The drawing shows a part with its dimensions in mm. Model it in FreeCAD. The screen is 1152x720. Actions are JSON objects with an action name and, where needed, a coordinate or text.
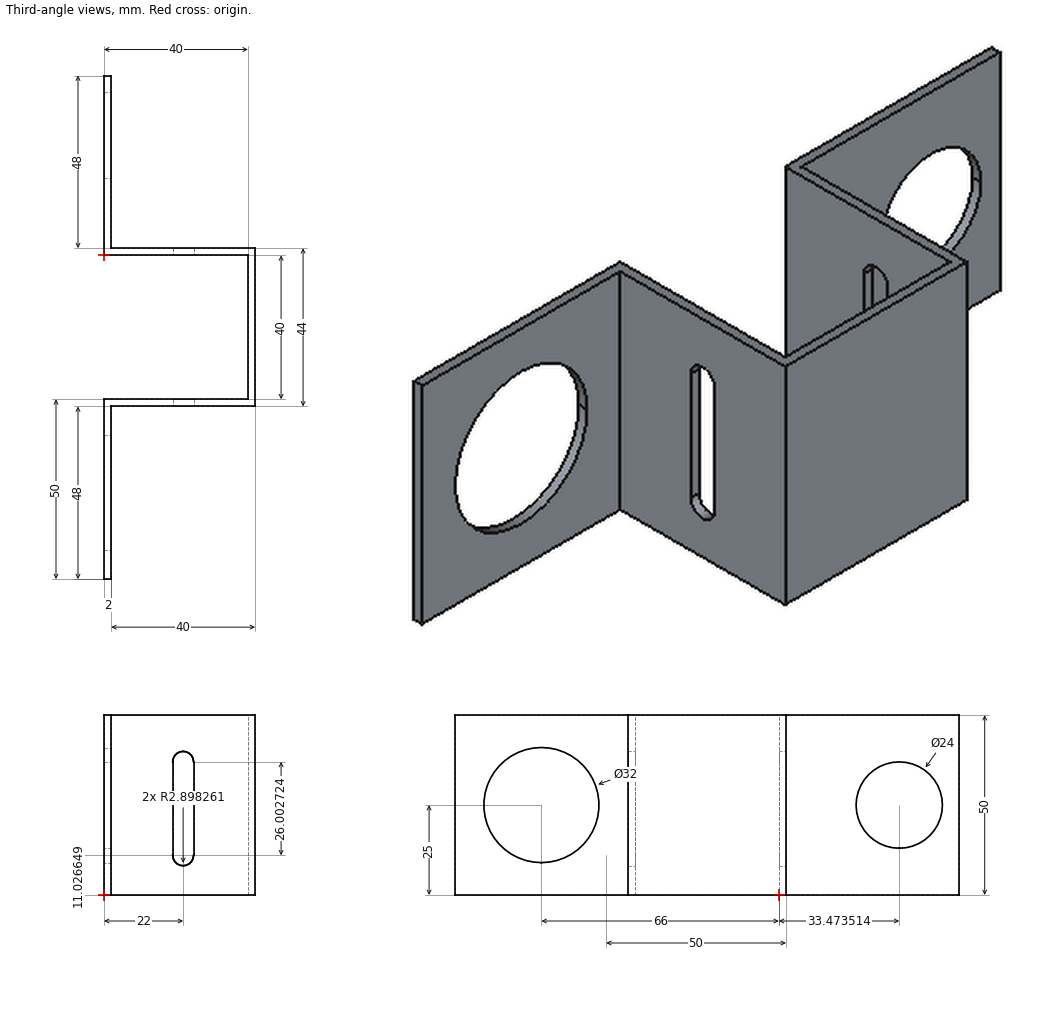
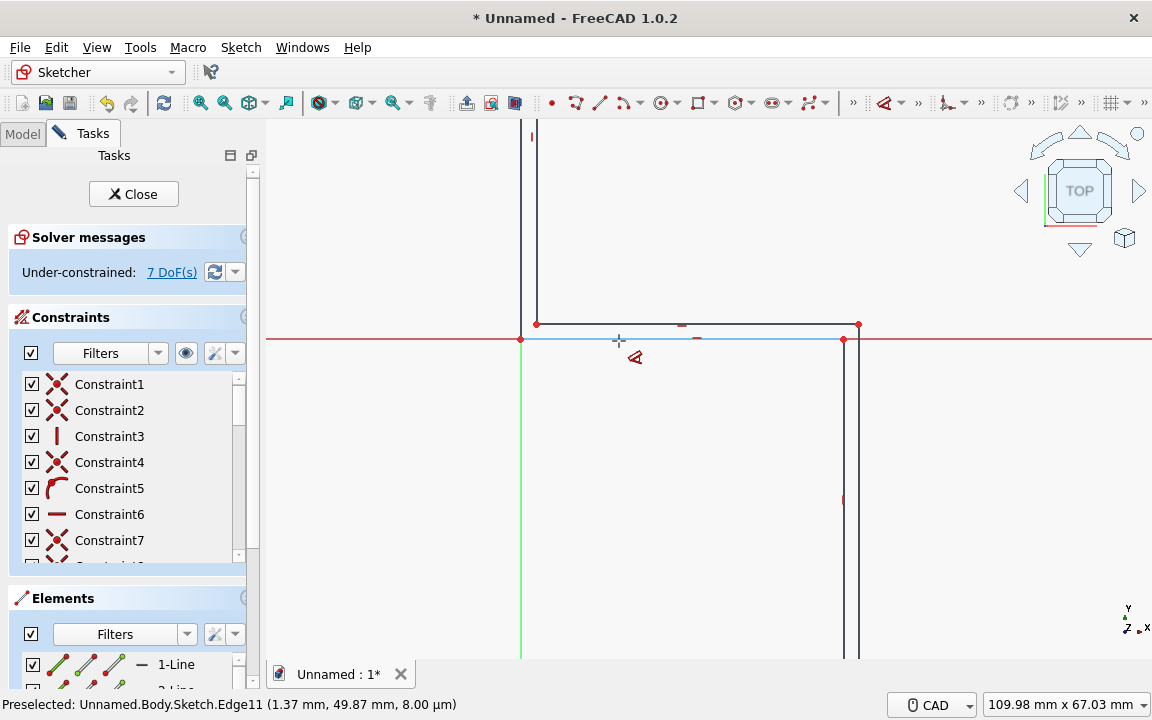
{"action": "left_click", "coordinate": [618, 339]}
{"action": "left_click", "coordinate": [682, 305]}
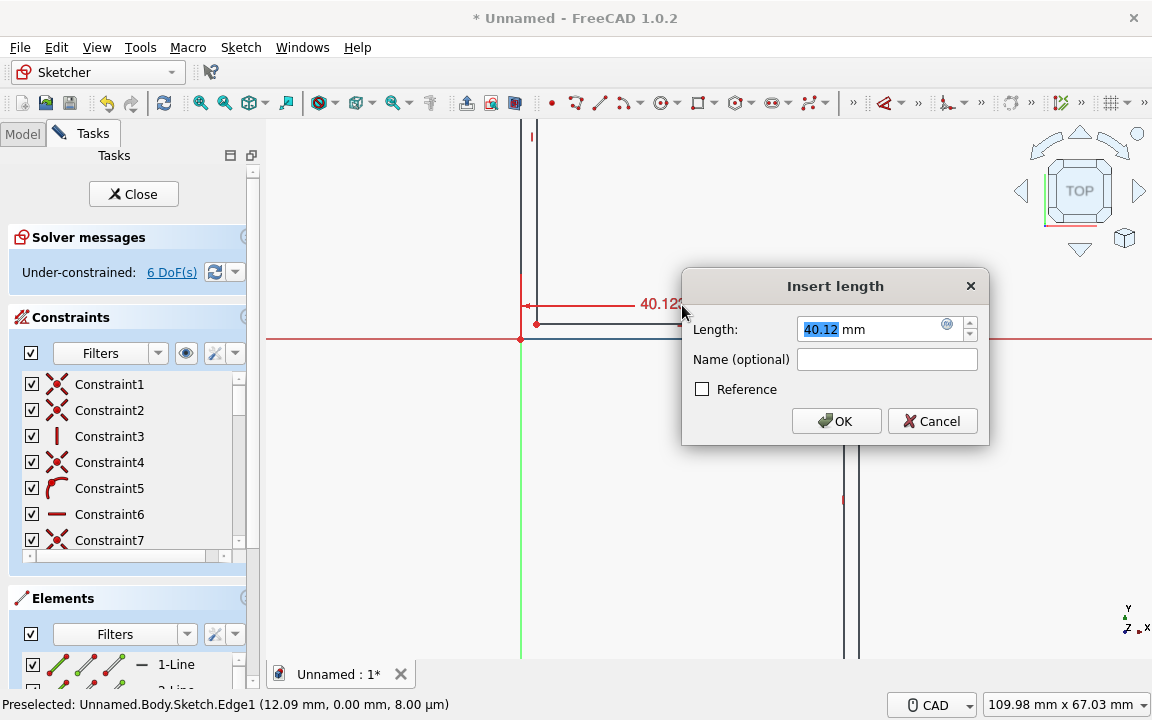
{"action": "type", "text": "40"}
{"action": "key", "text": "Return"}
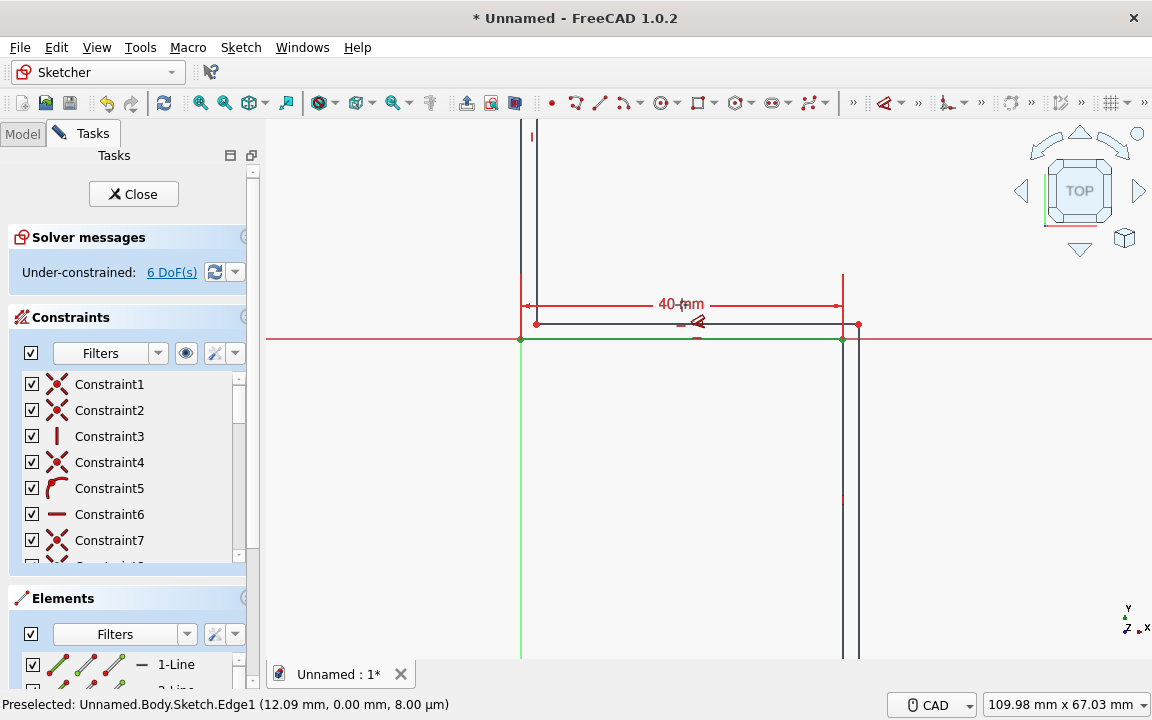
{"action": "left_click", "coordinate": [843, 437]}
{"action": "left_click", "coordinate": [877, 485]}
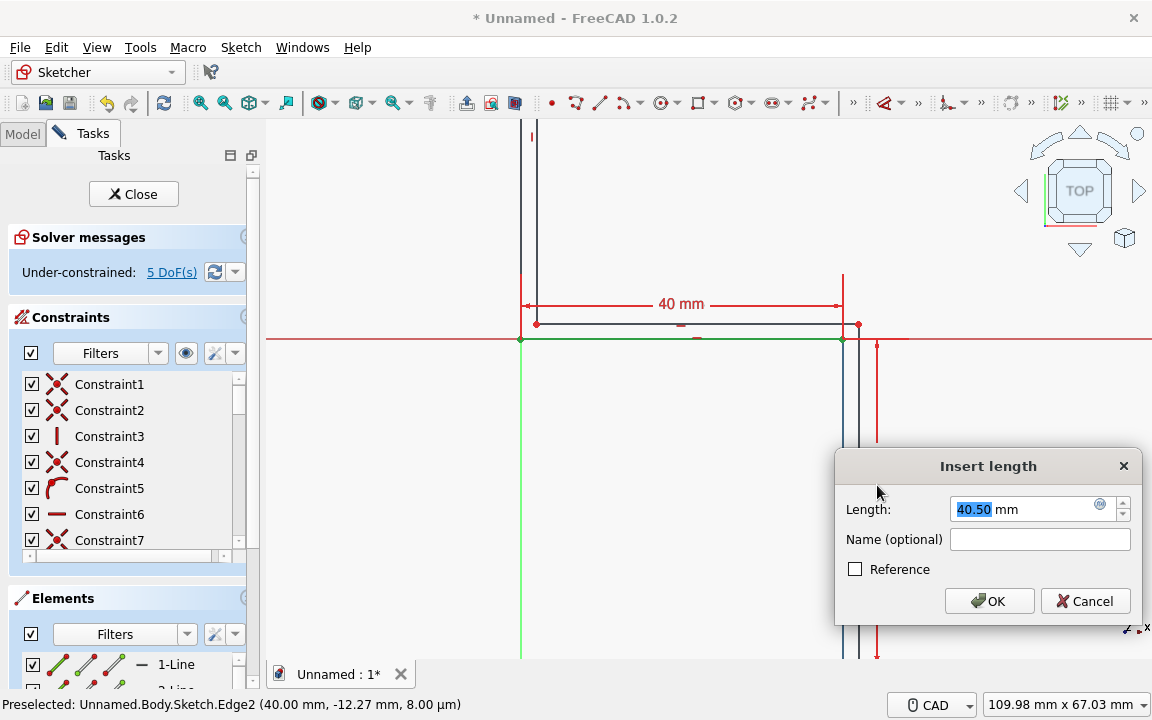
{"action": "type", "text": "40"}
{"action": "key", "text": "Return"}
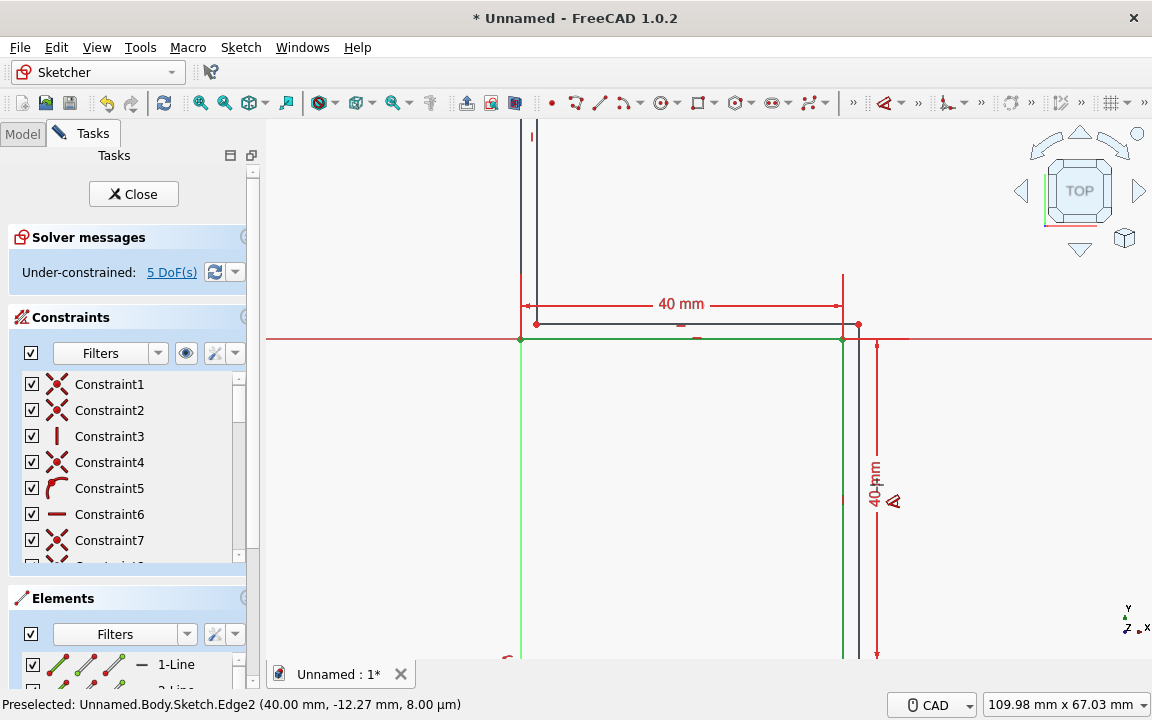
{"action": "scroll", "coordinate": [619, 341], "scroll_direction": "down", "scroll_amount": 6}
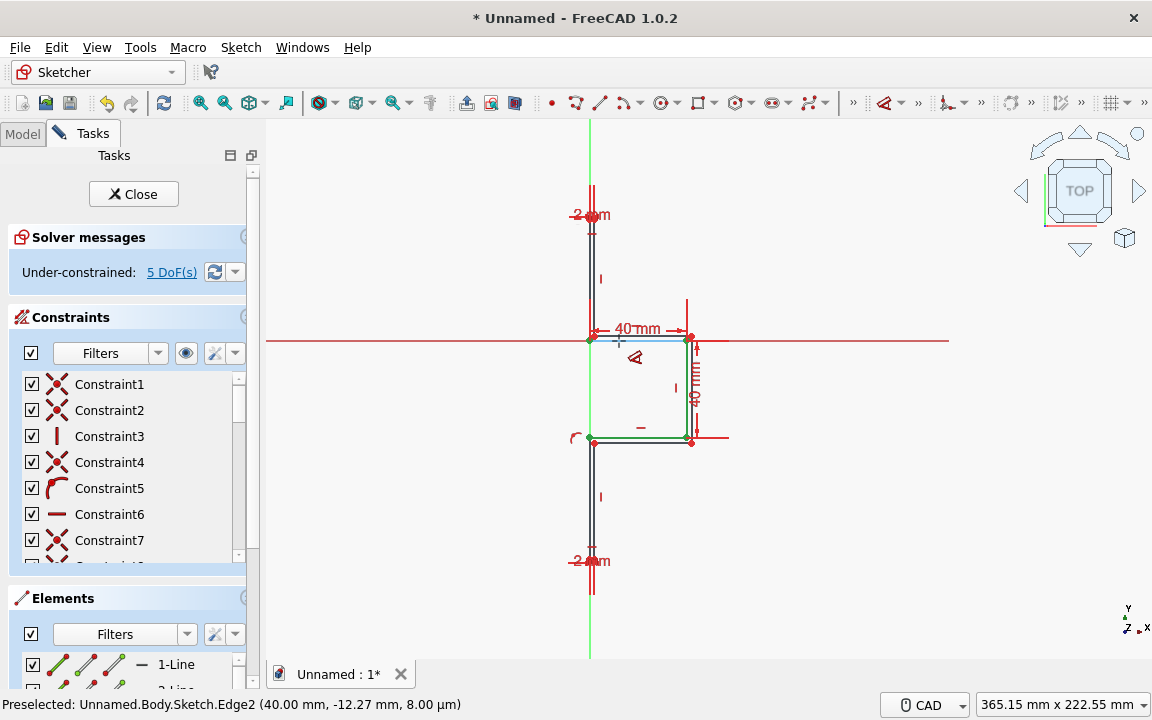
{"action": "scroll", "coordinate": [590, 474], "scroll_direction": "up", "scroll_amount": 6}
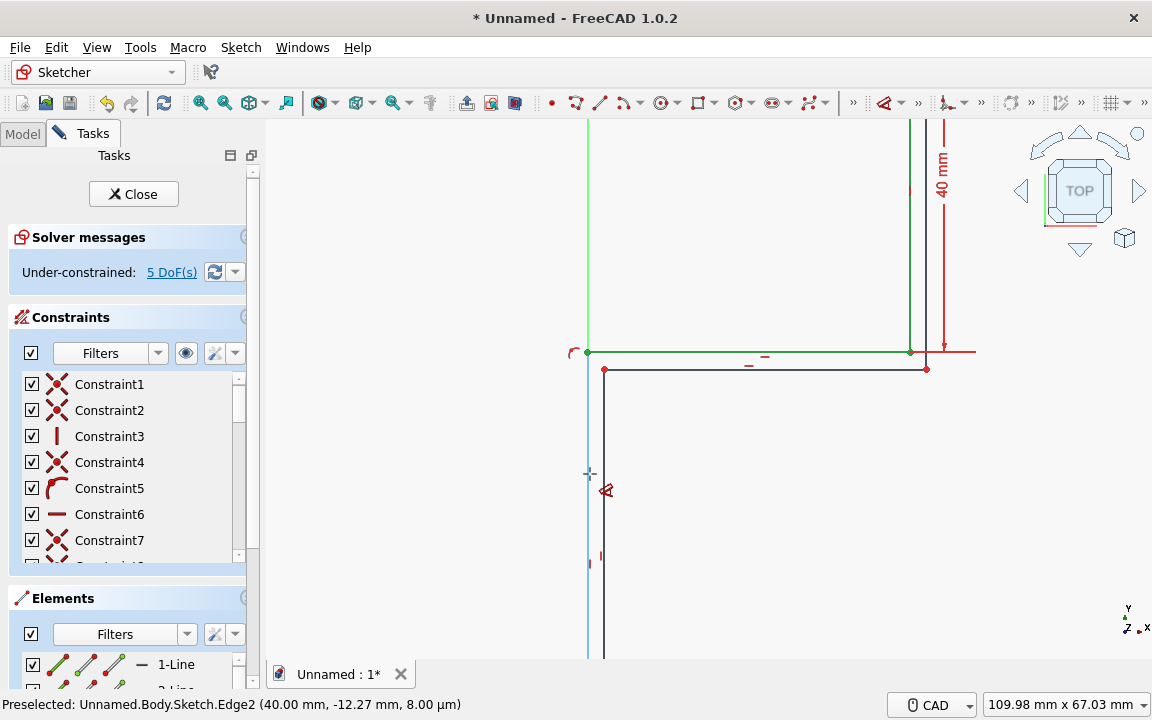
{"action": "left_click", "coordinate": [588, 474]}
{"action": "left_click", "coordinate": [554, 492]}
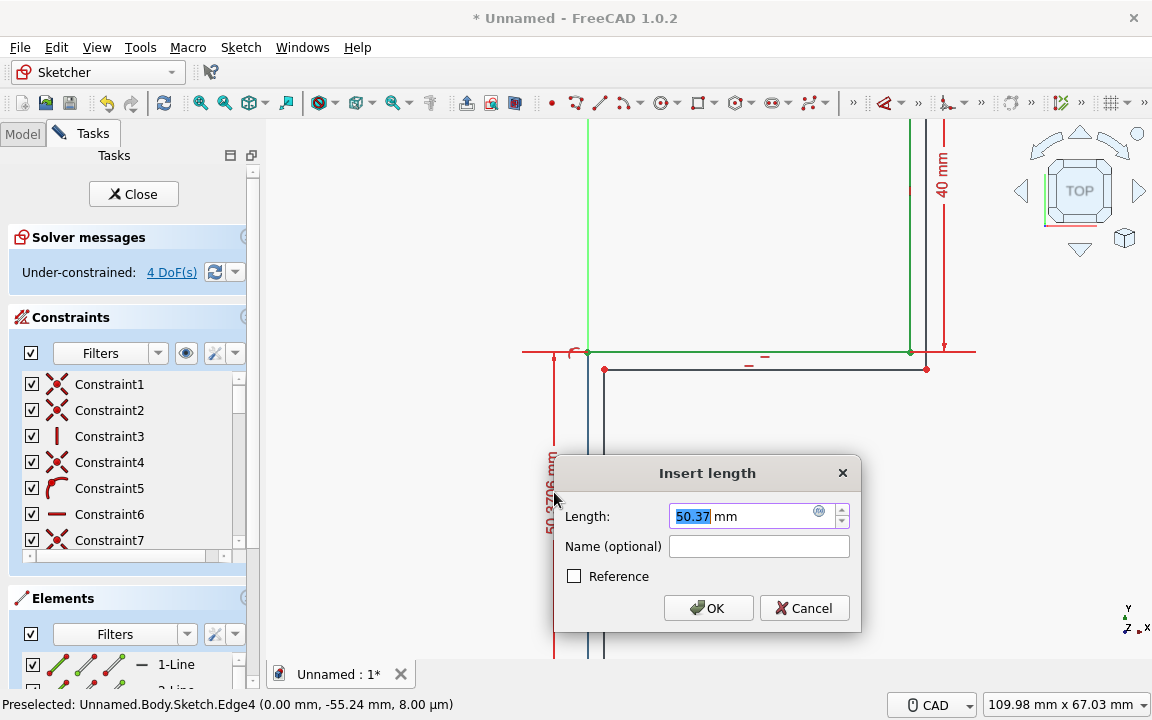
{"action": "type", "text": "50"}
{"action": "key", "text": "Return"}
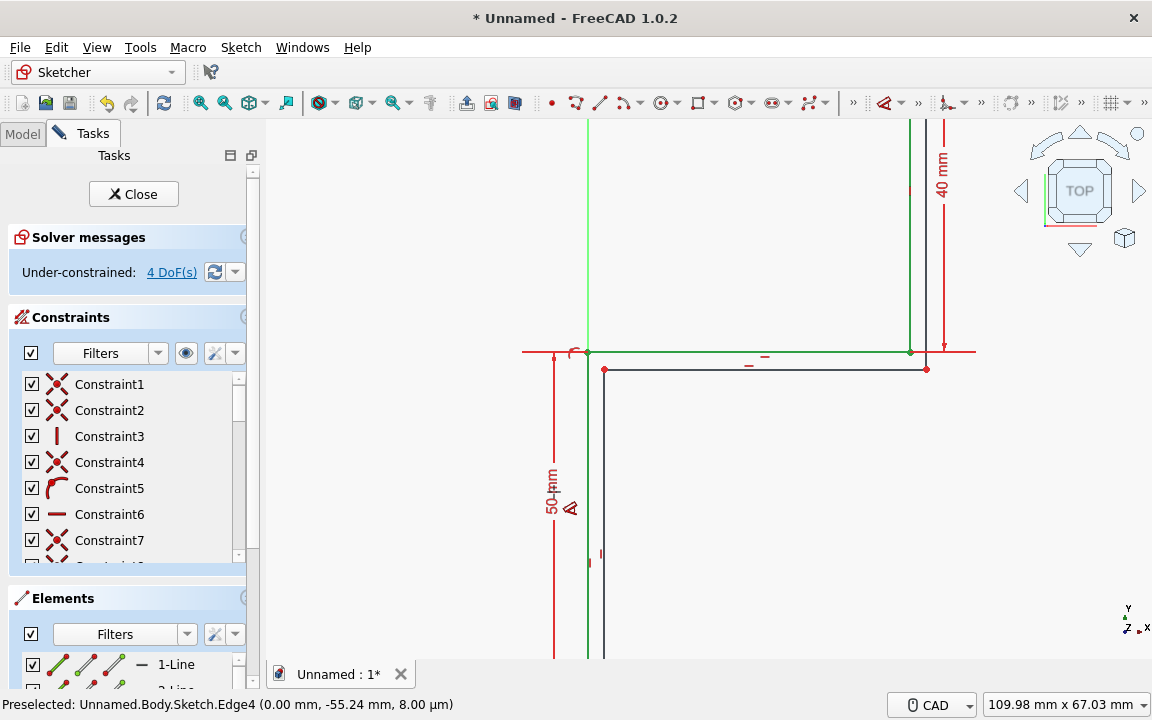
{"action": "left_click", "coordinate": [604, 485]}
{"action": "left_click", "coordinate": [570, 440]}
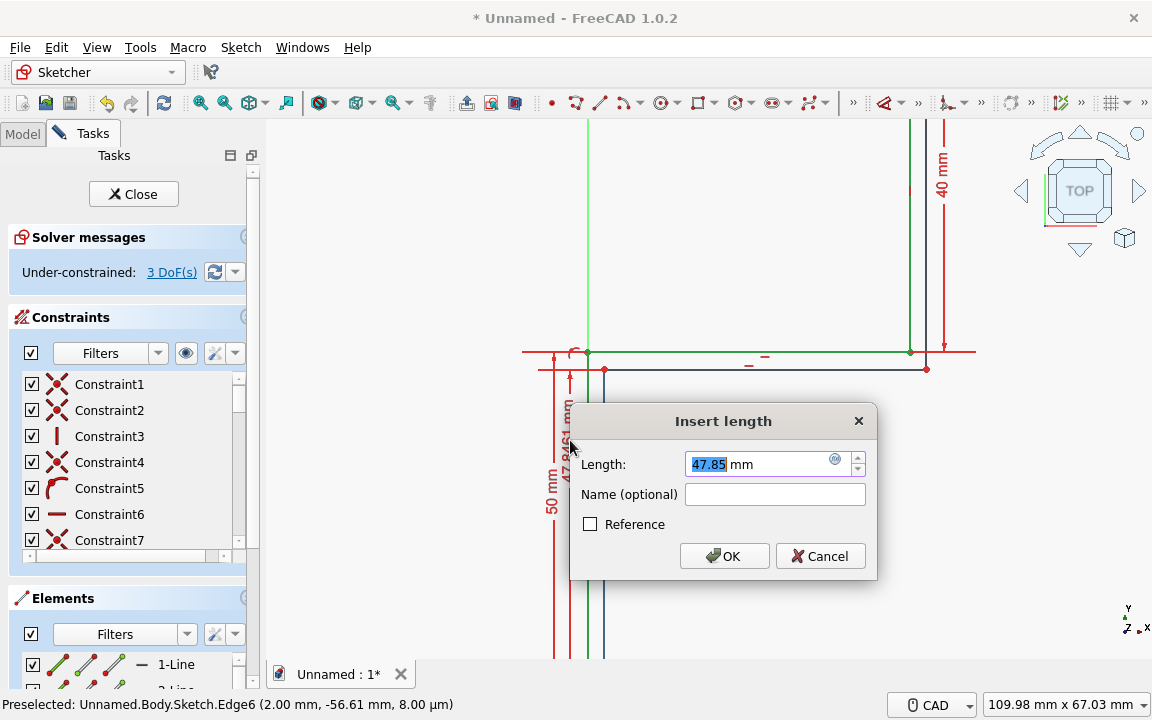
{"action": "type", "text": "48"}
{"action": "key", "text": "Return"}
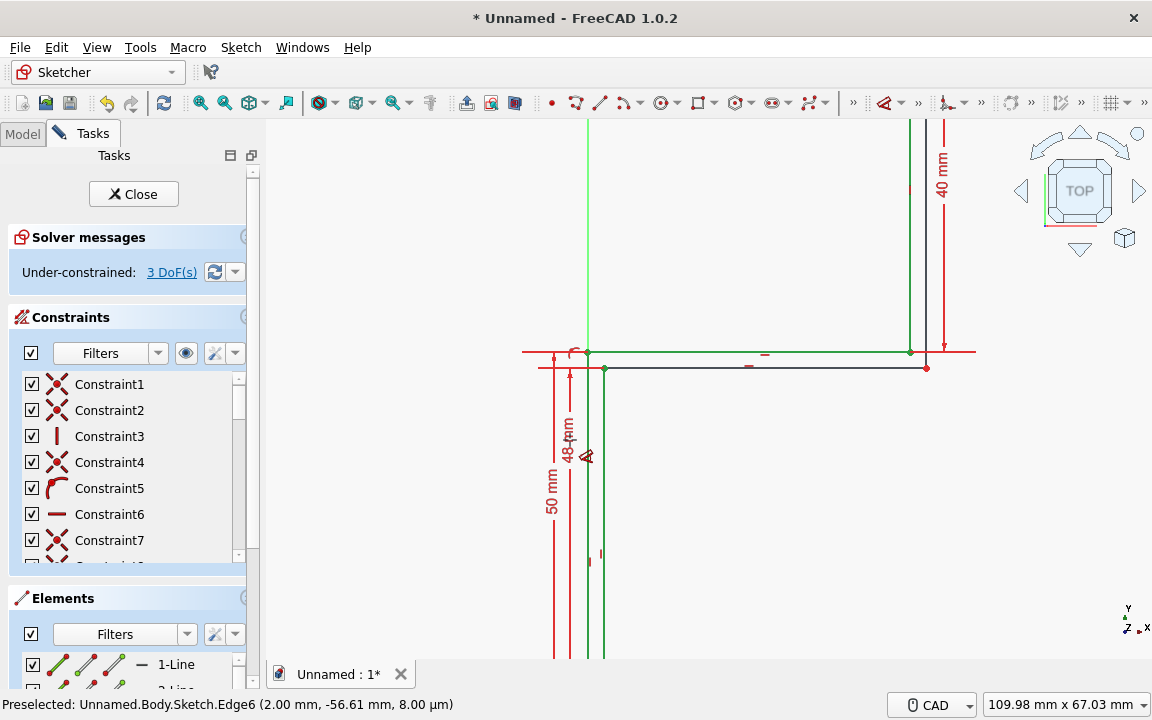
{"action": "left_click", "coordinate": [701, 368]}
{"action": "left_click", "coordinate": [765, 402]}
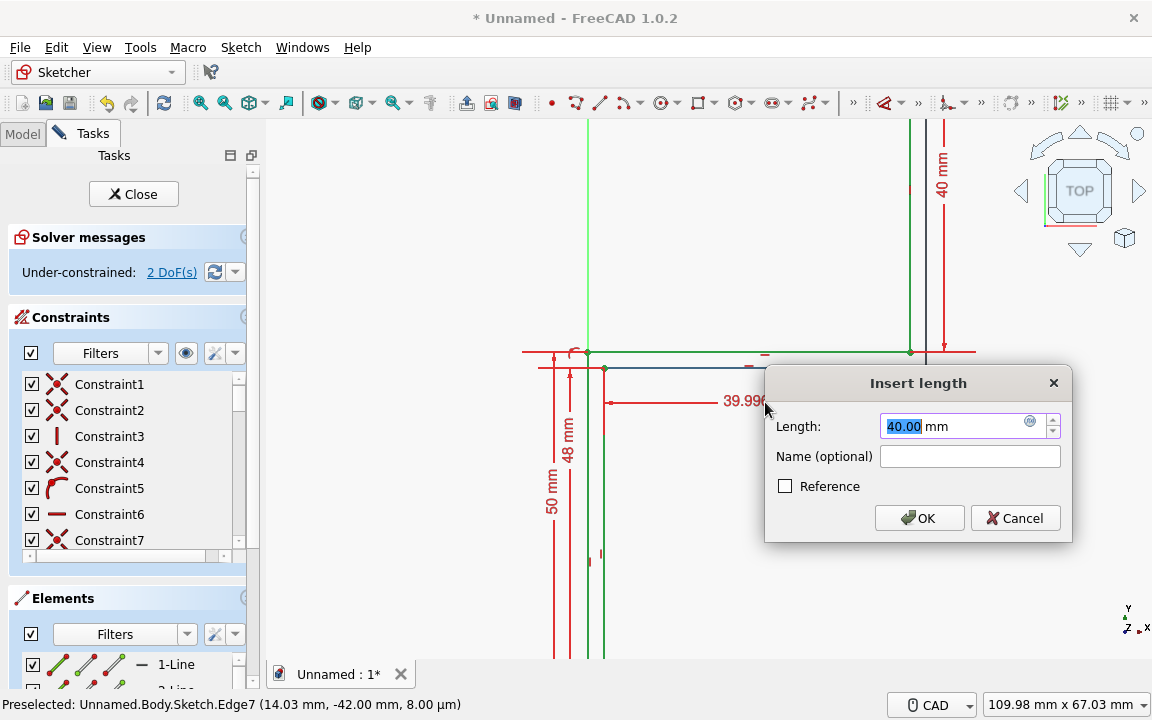
{"action": "type", "text": "40"}
{"action": "key", "text": "Return"}